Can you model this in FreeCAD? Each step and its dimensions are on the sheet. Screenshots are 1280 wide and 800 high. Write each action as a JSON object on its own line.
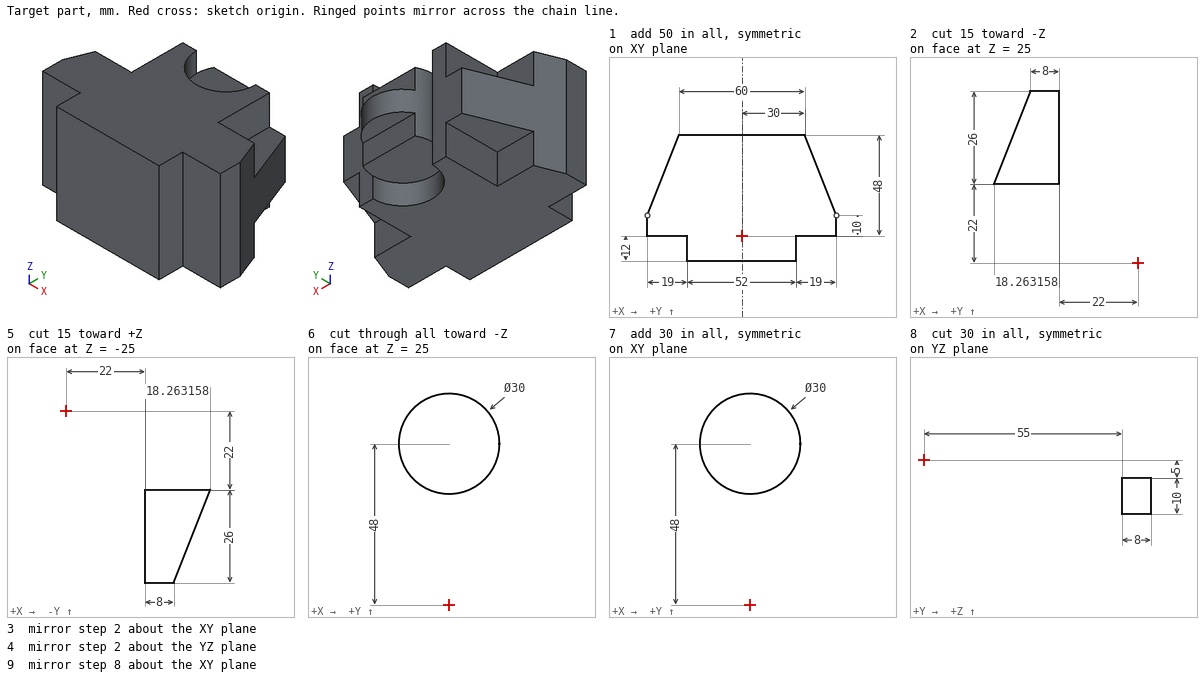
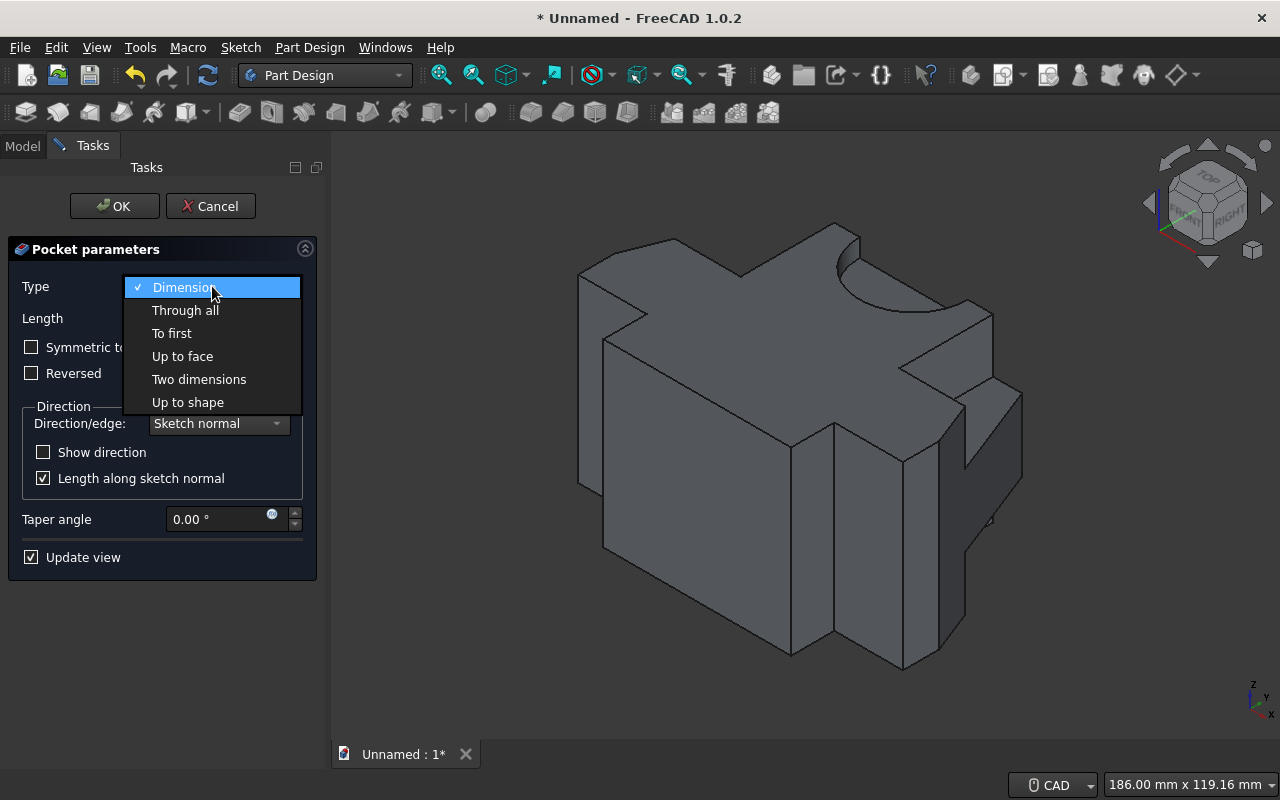
{"action": "left_click", "coordinate": [212, 310]}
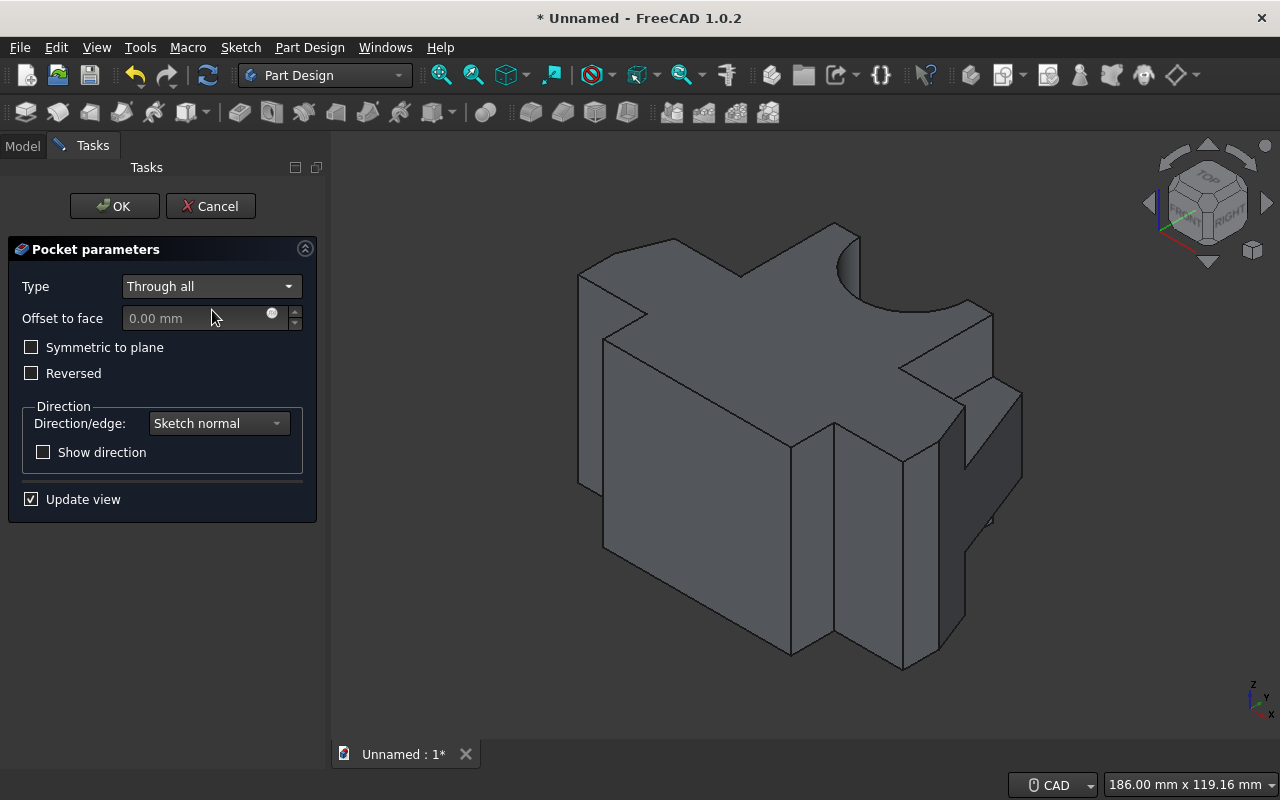
{"action": "left_click", "coordinate": [115, 206]}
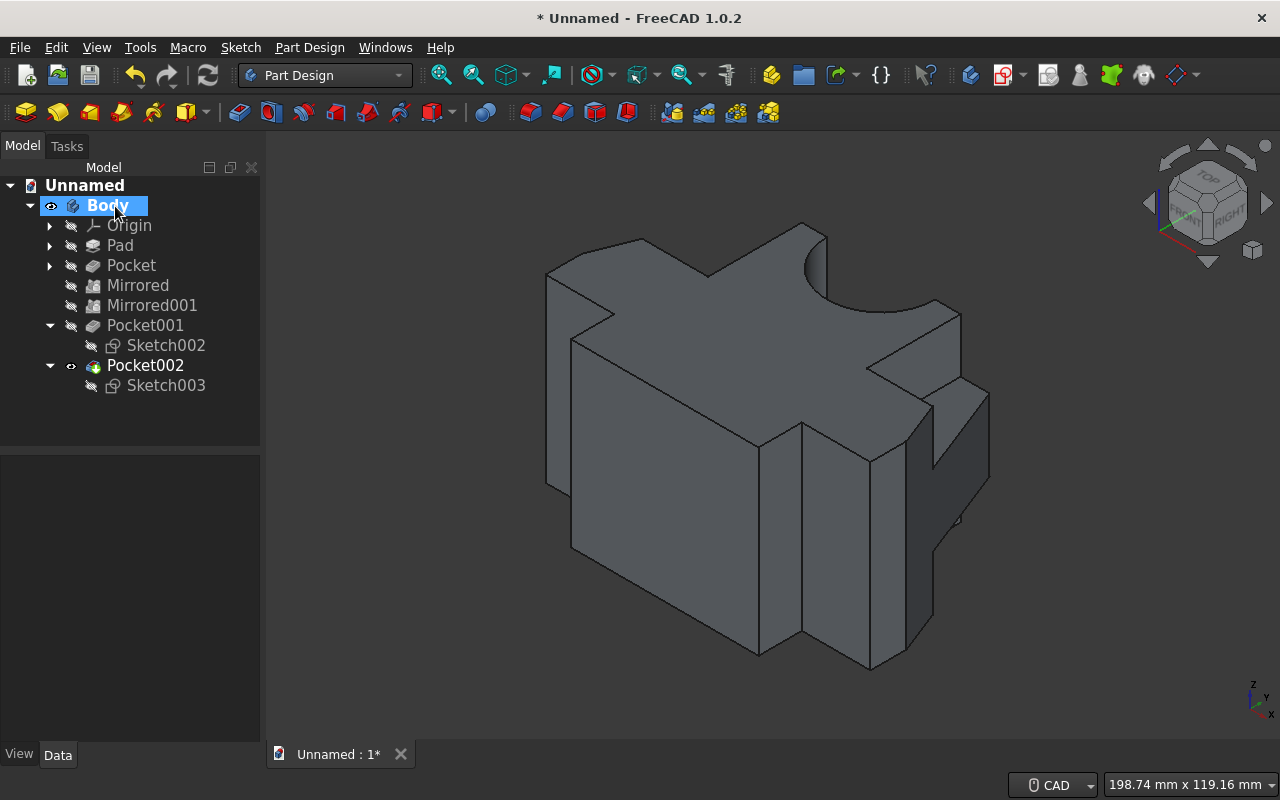
{"action": "left_click", "coordinate": [1004, 76]}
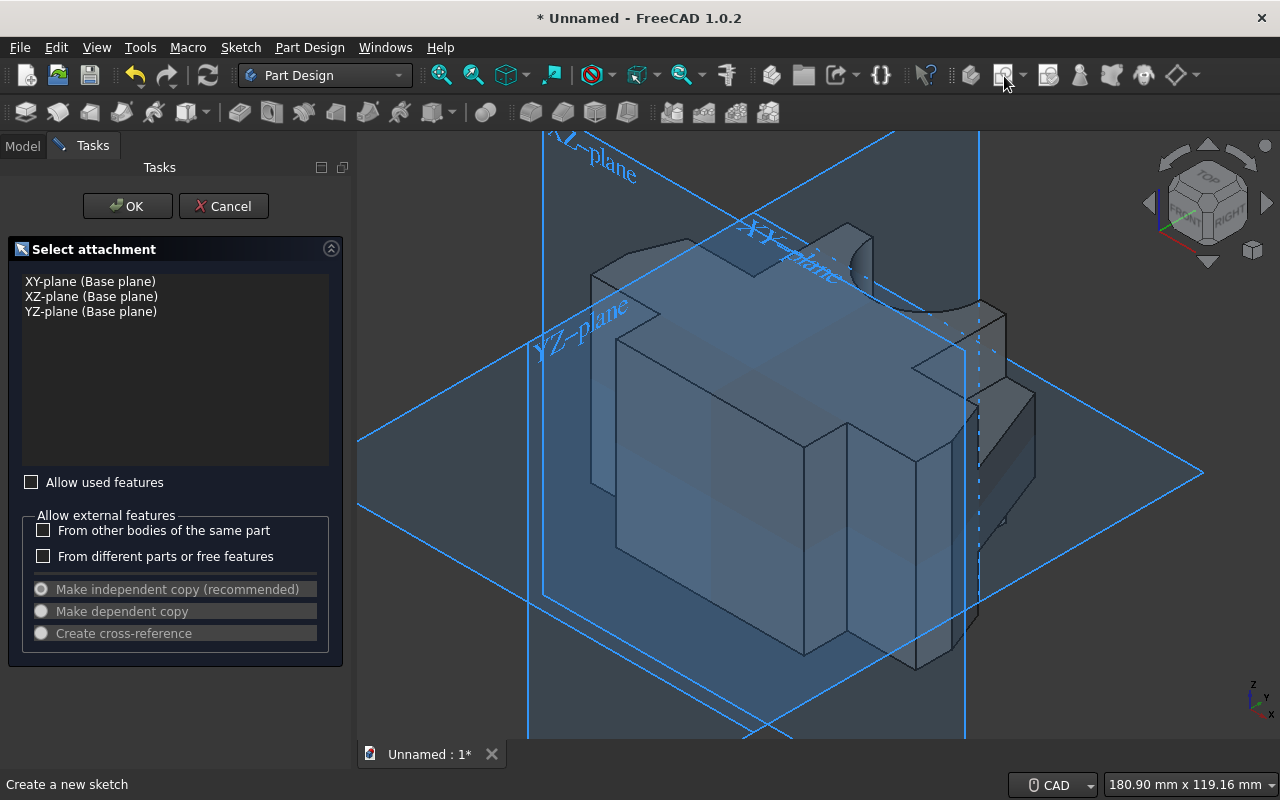
{"action": "left_click", "coordinate": [82, 282]}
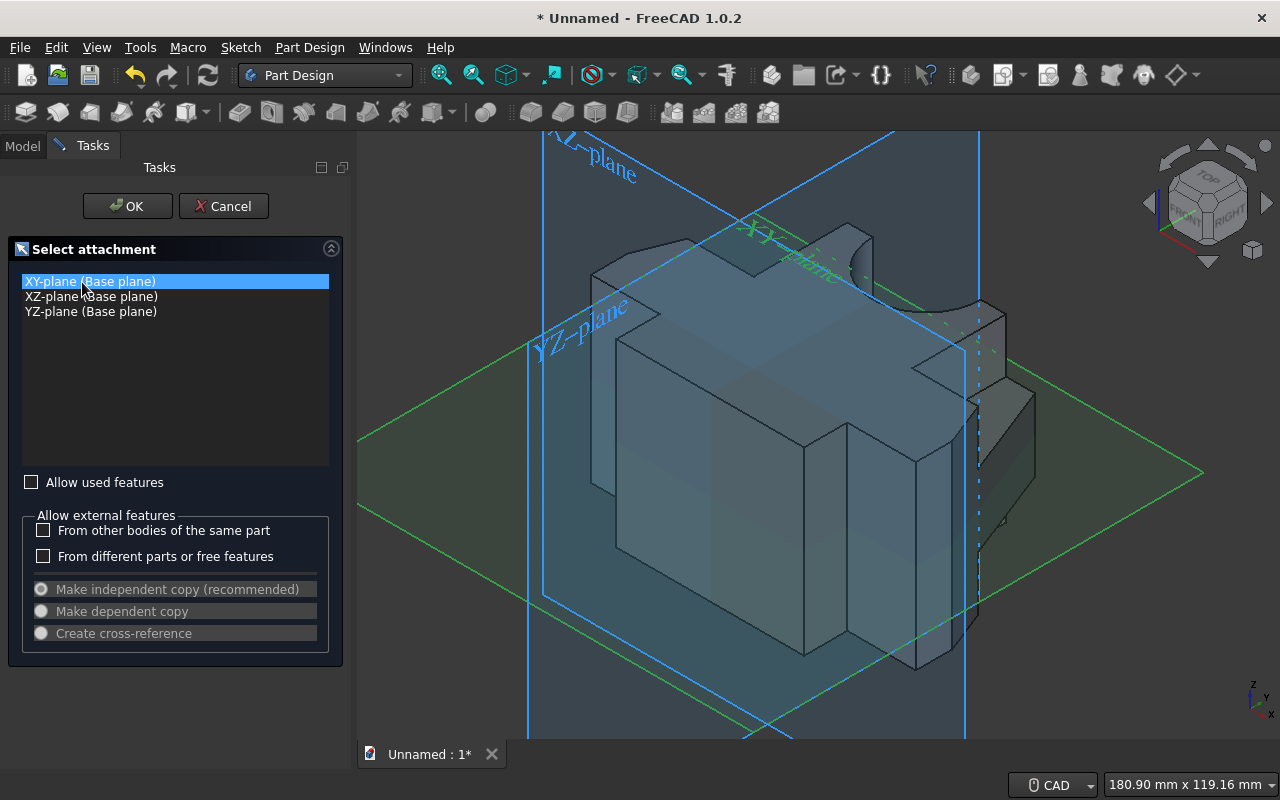
{"action": "left_click", "coordinate": [128, 206]}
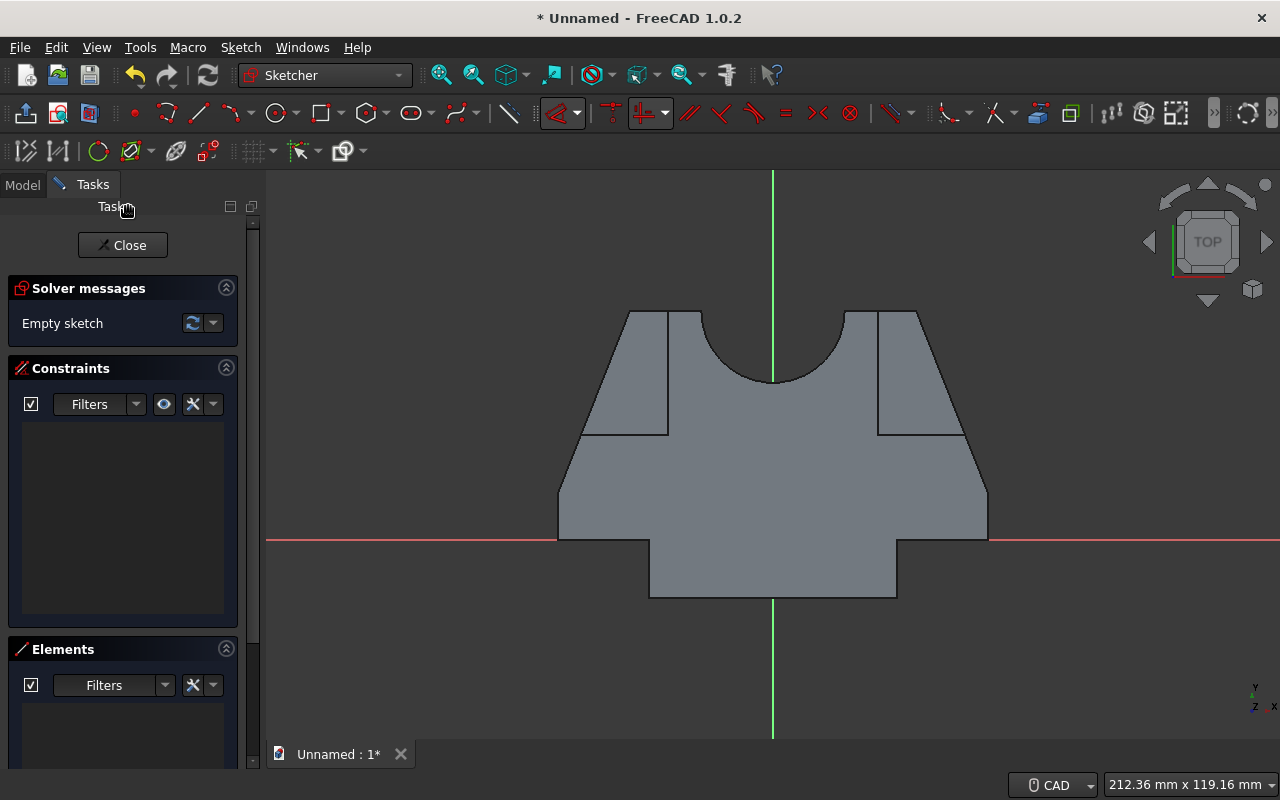
{"action": "left_click", "coordinate": [90, 114]}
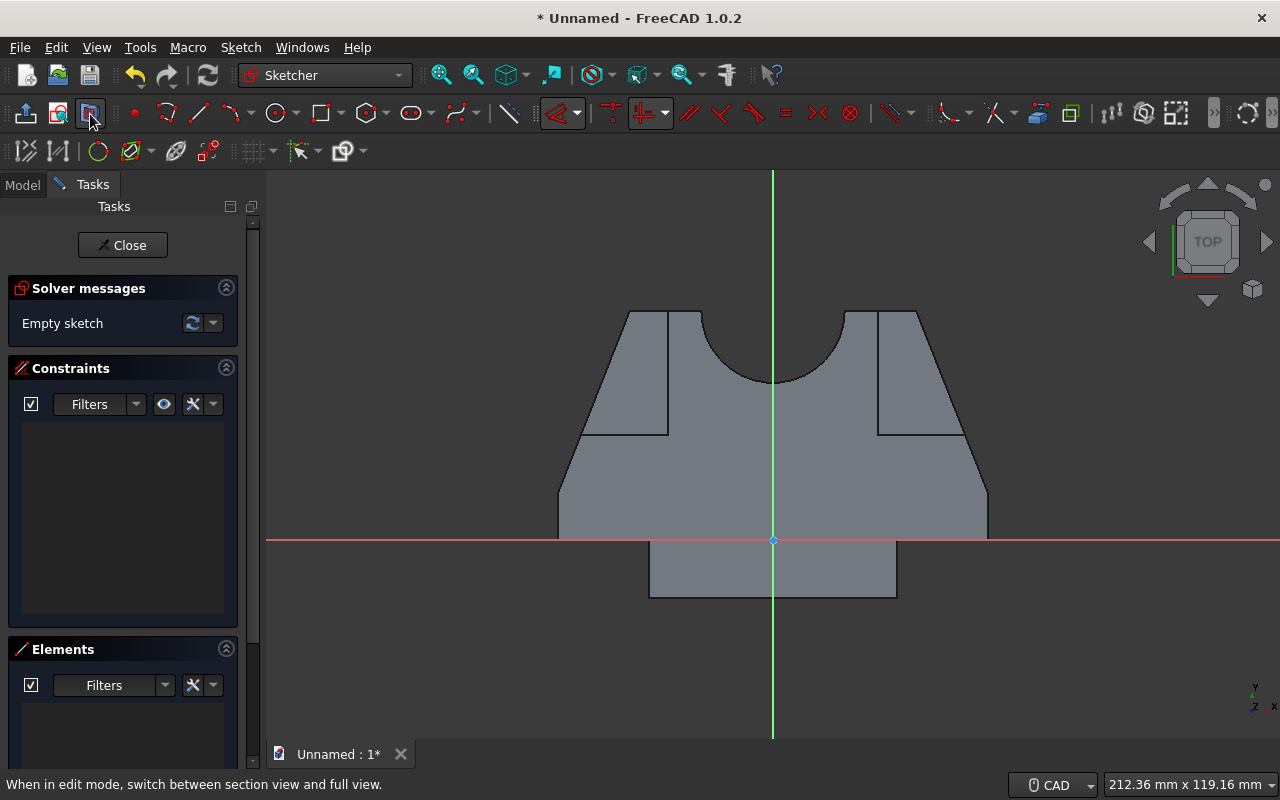
{"action": "left_click", "coordinate": [276, 114]}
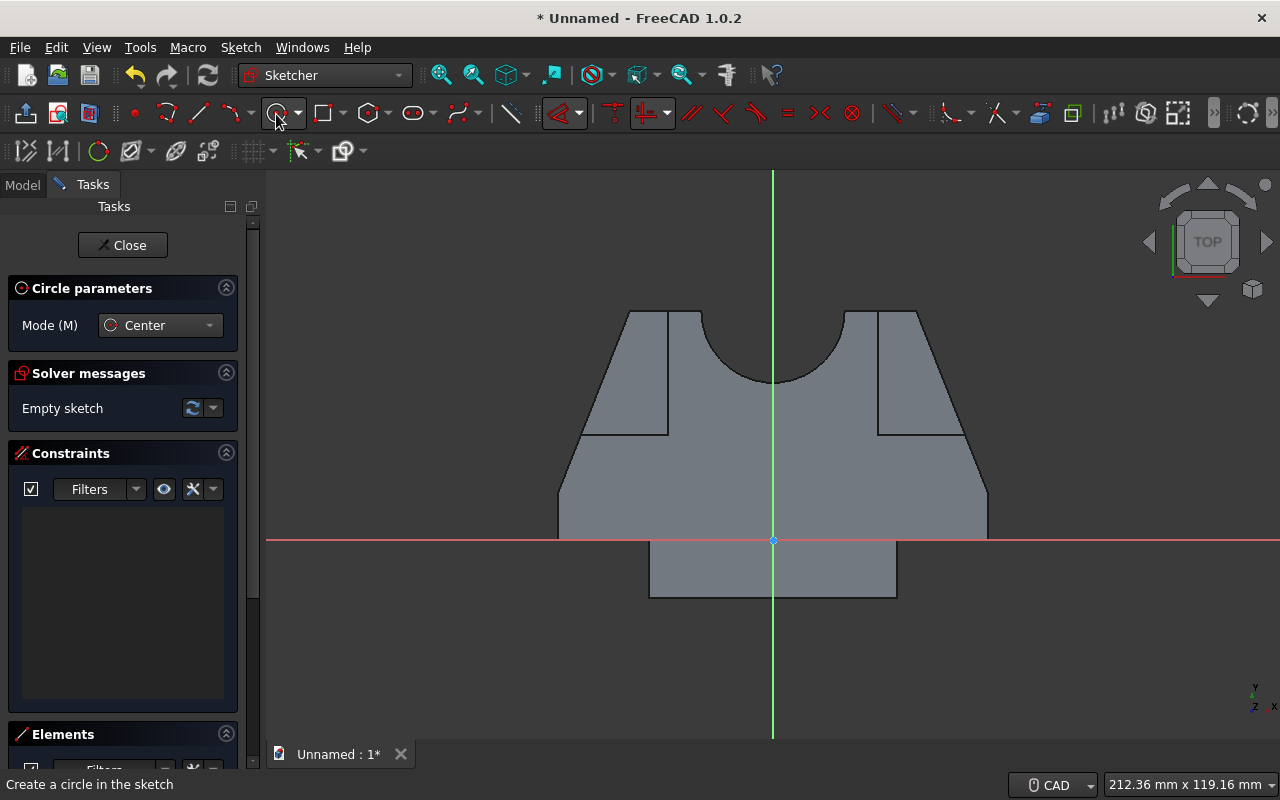
{"action": "left_click", "coordinate": [773, 311]}
{"action": "left_click", "coordinate": [824, 261]}
{"action": "key", "text": "Escape"}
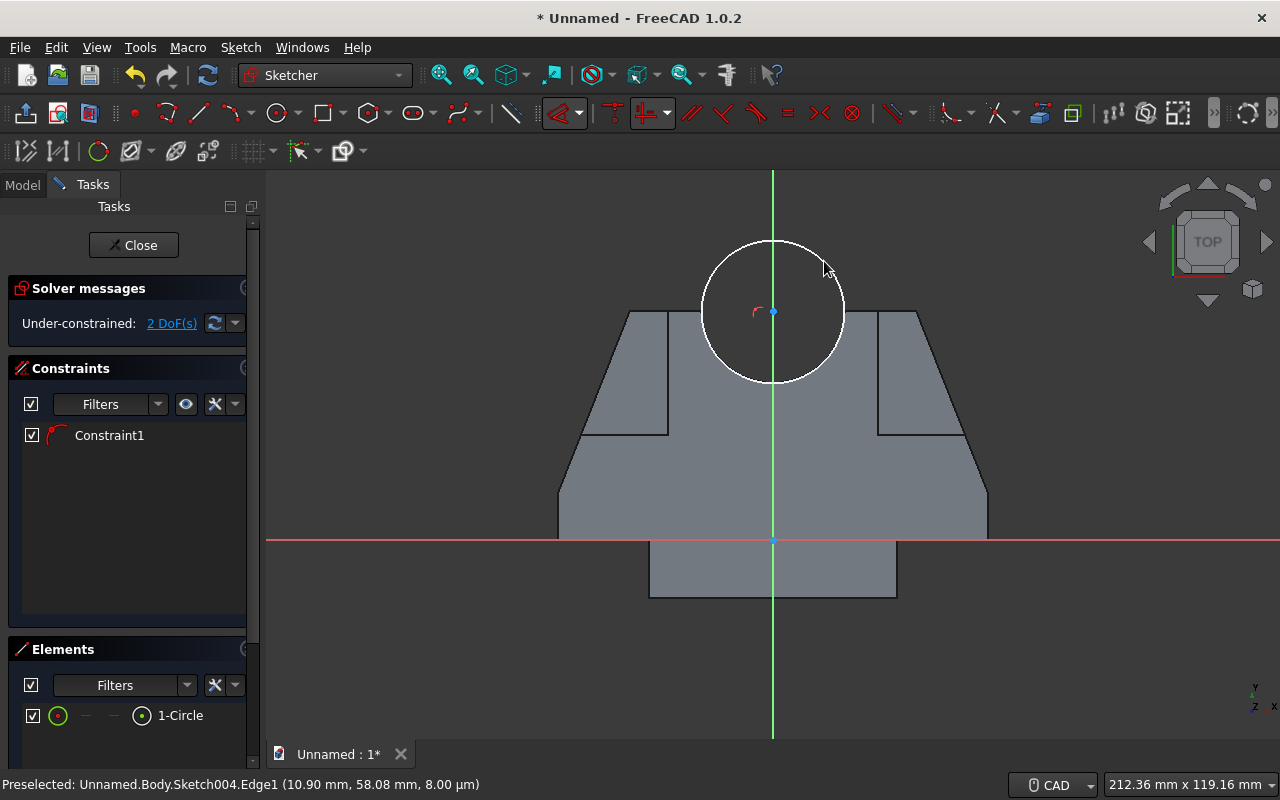
{"action": "left_click", "coordinate": [823, 261]}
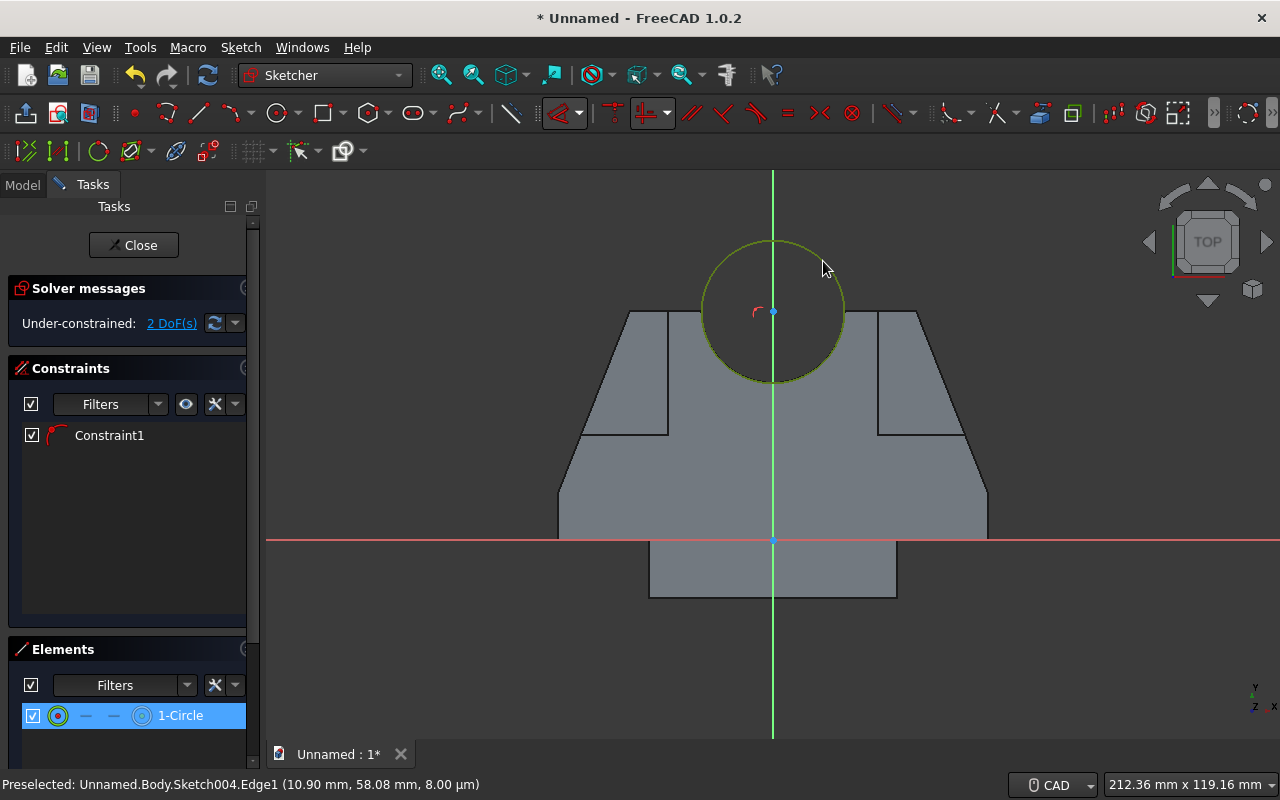
{"action": "left_click", "coordinate": [582, 114]}